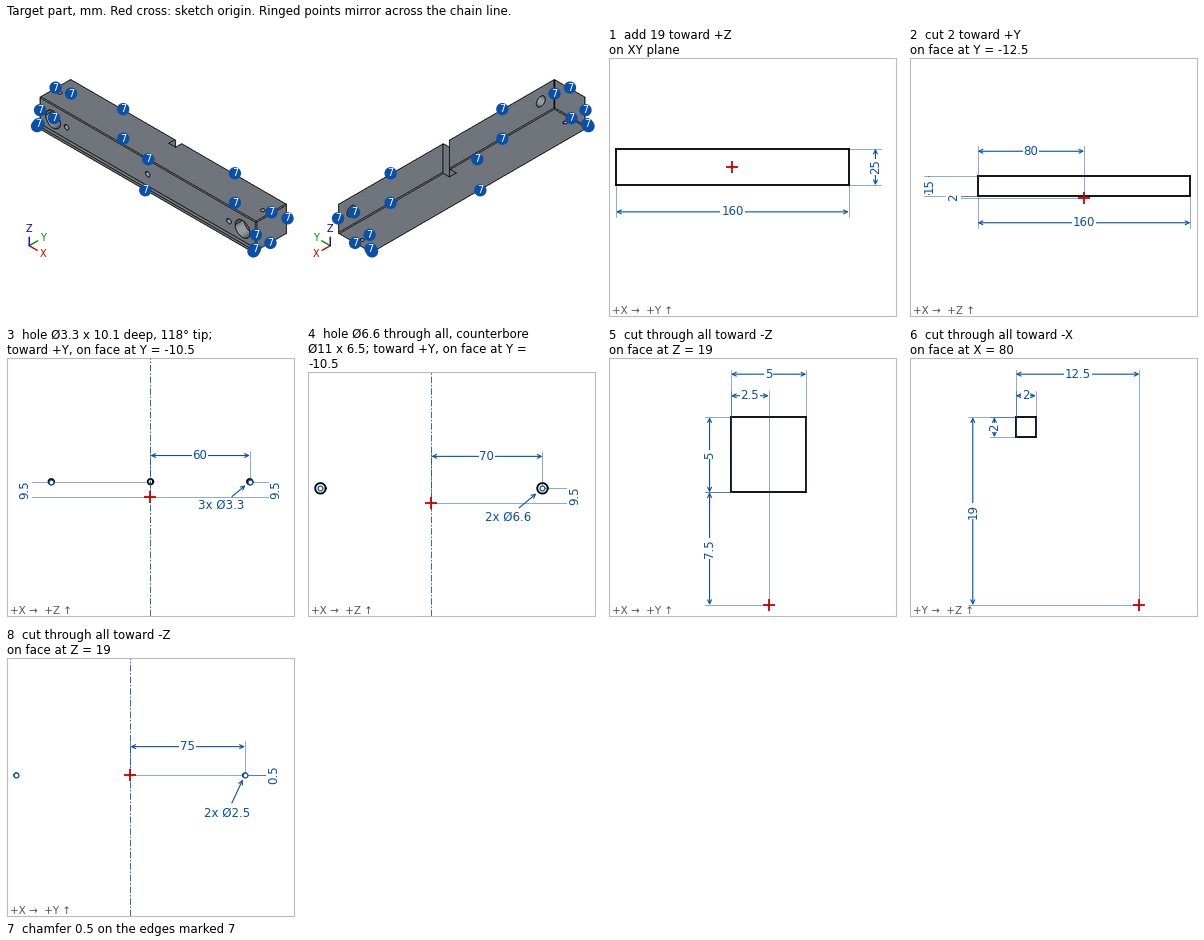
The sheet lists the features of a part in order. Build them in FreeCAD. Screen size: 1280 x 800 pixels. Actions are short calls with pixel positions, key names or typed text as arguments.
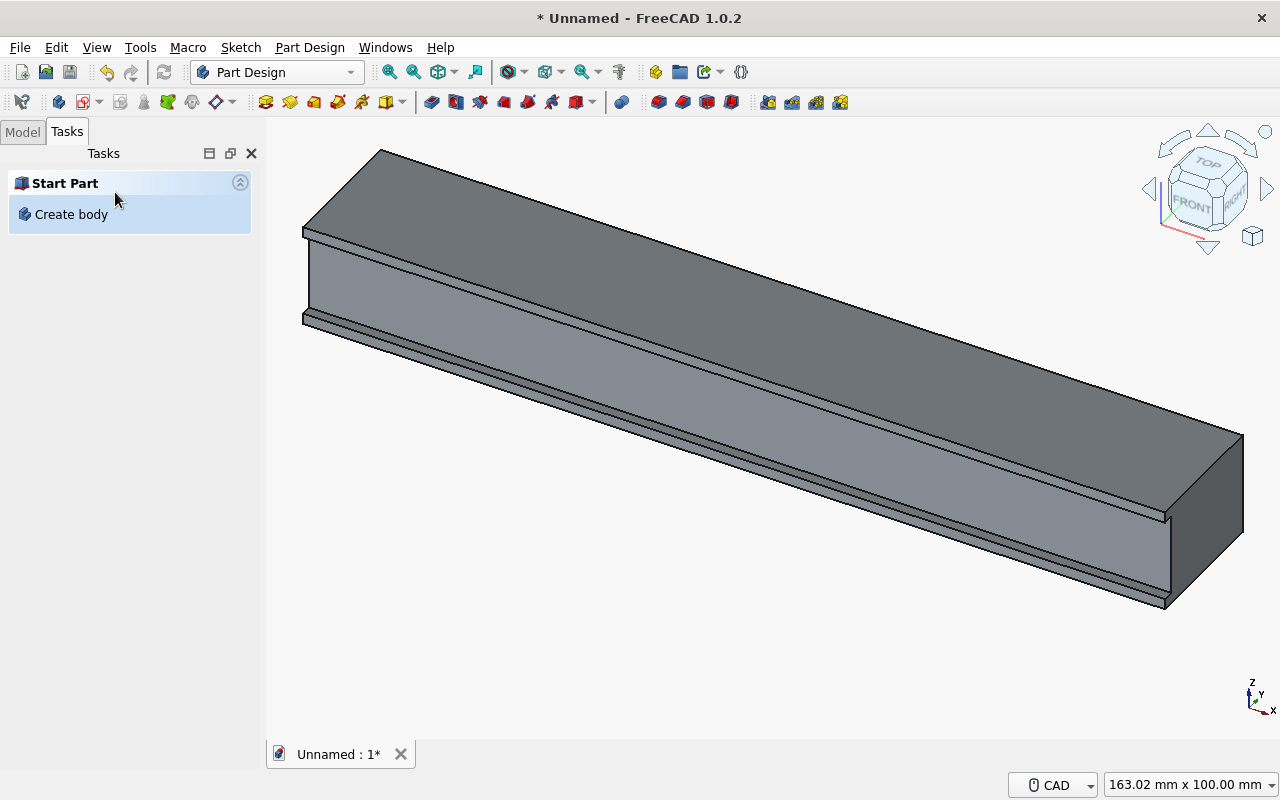
click(1110, 533)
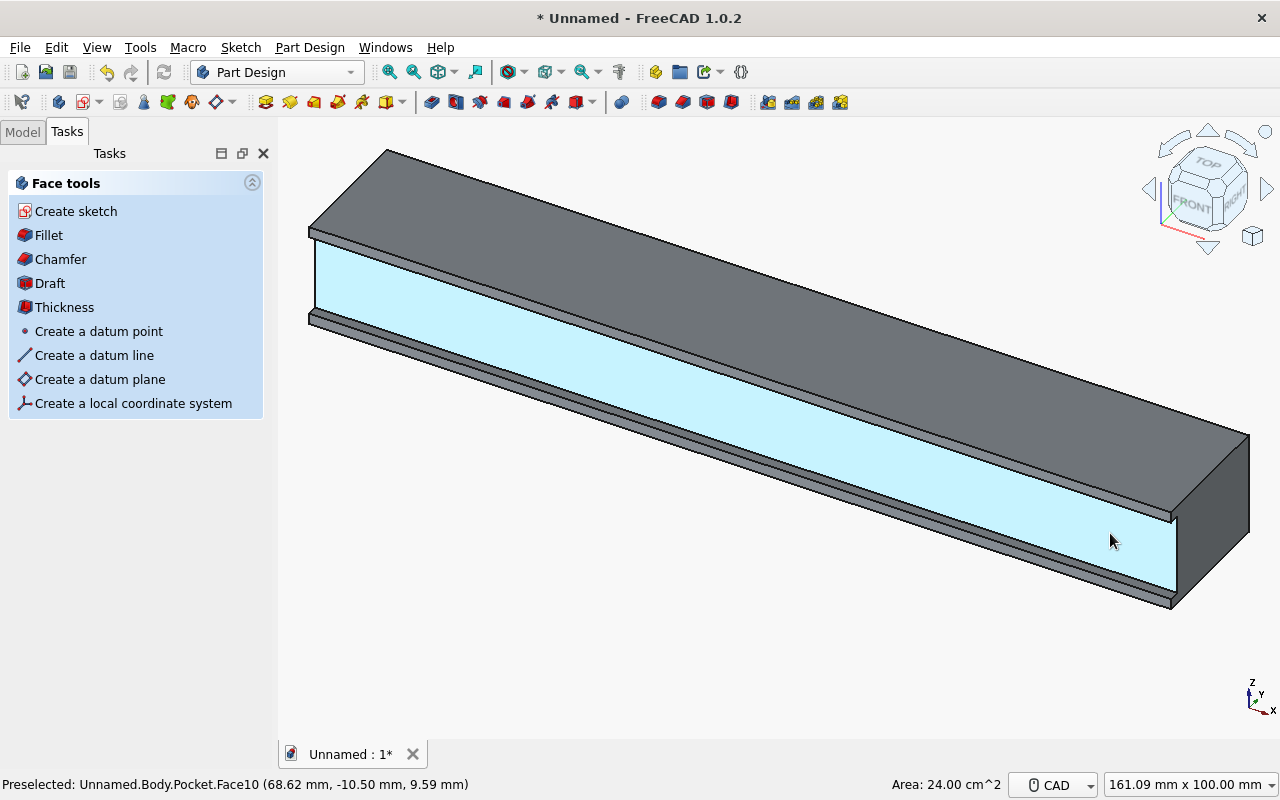
click(84, 102)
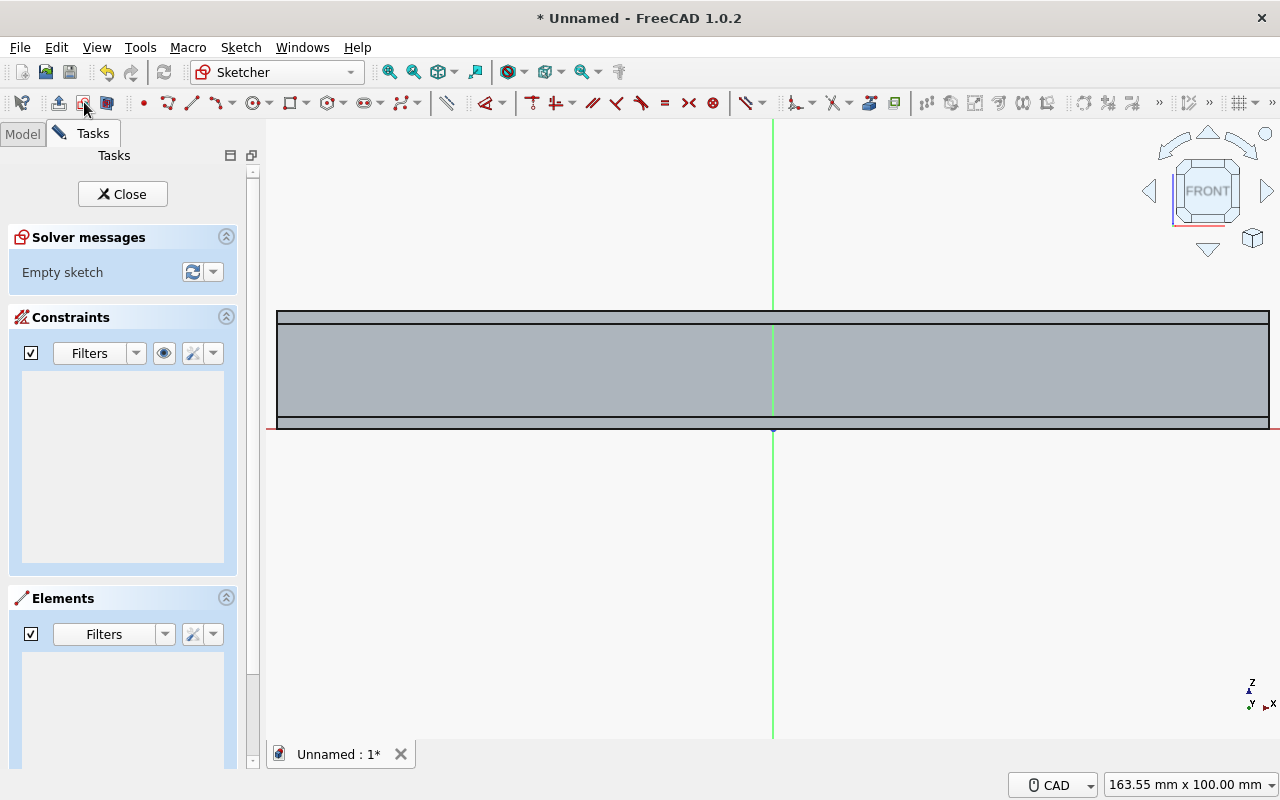
scroll(395, 585, down, 1)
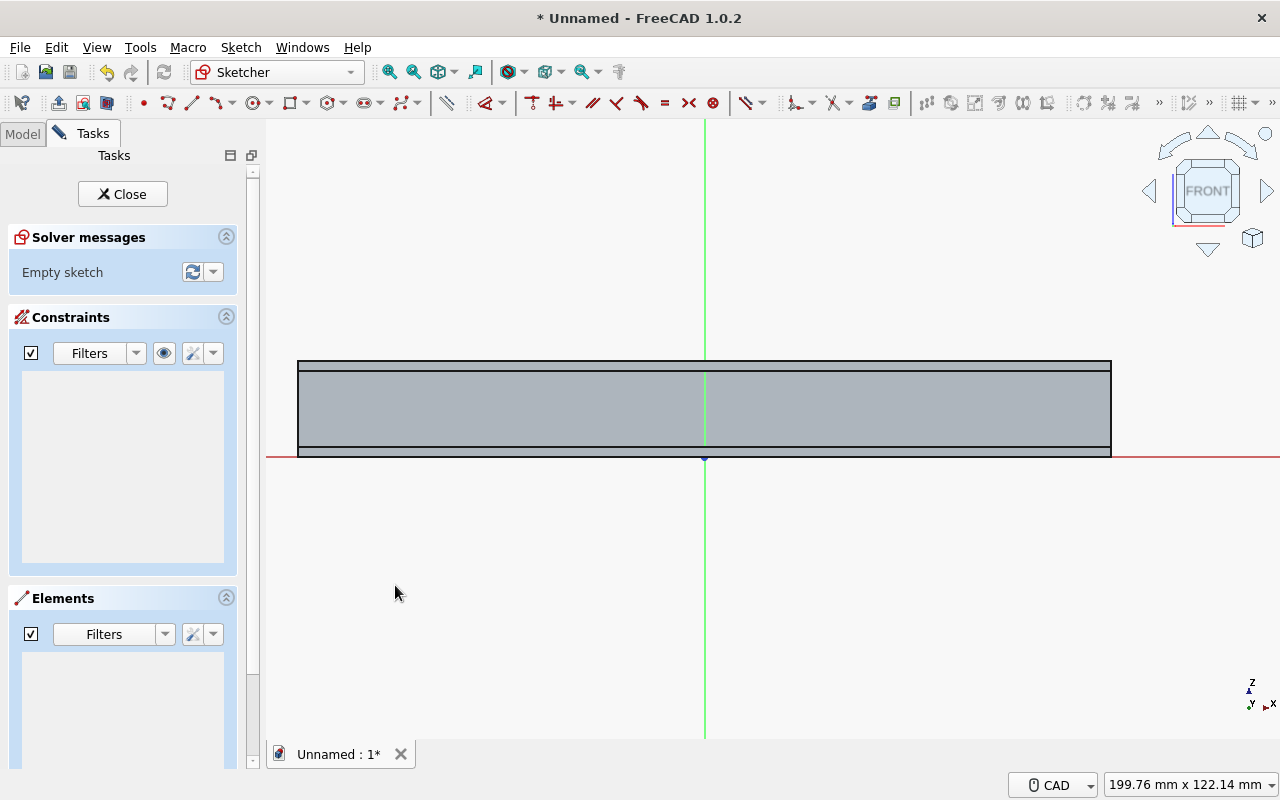
click(254, 104)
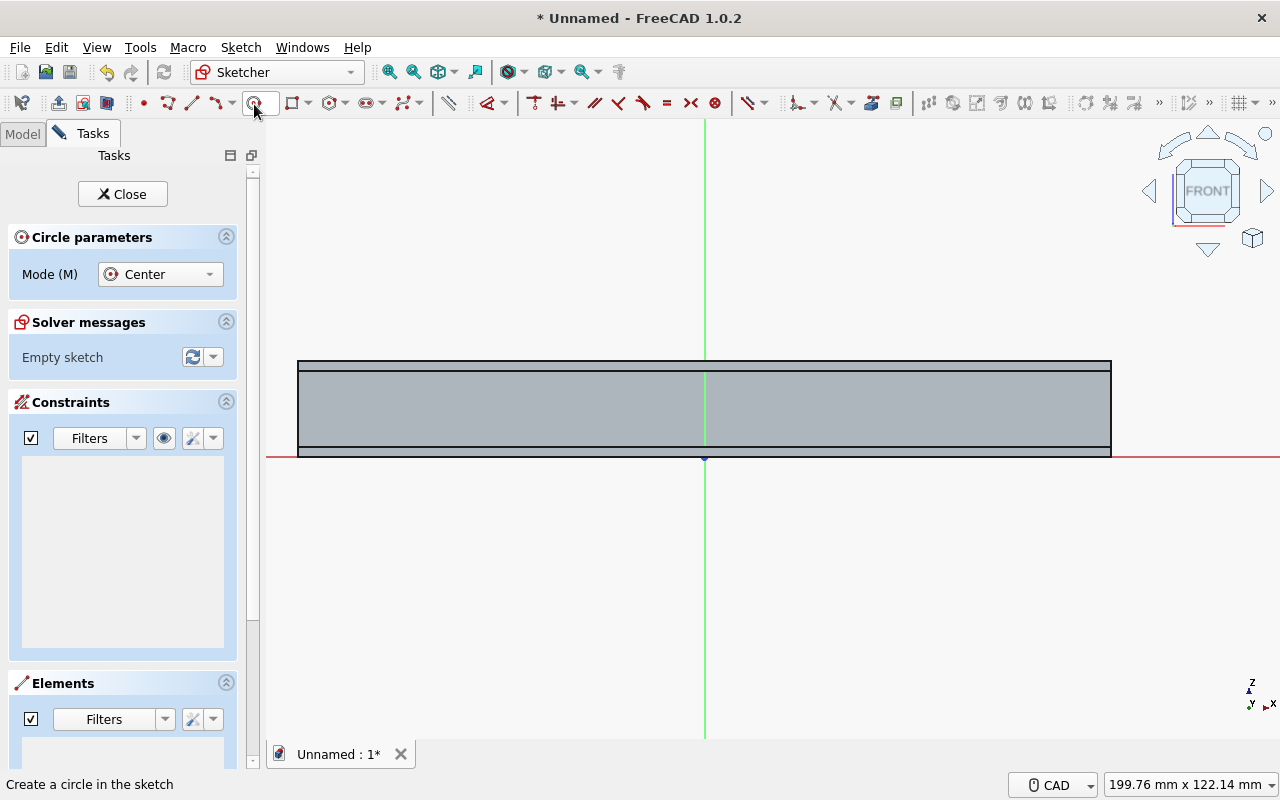
scroll(1009, 409, up, 5)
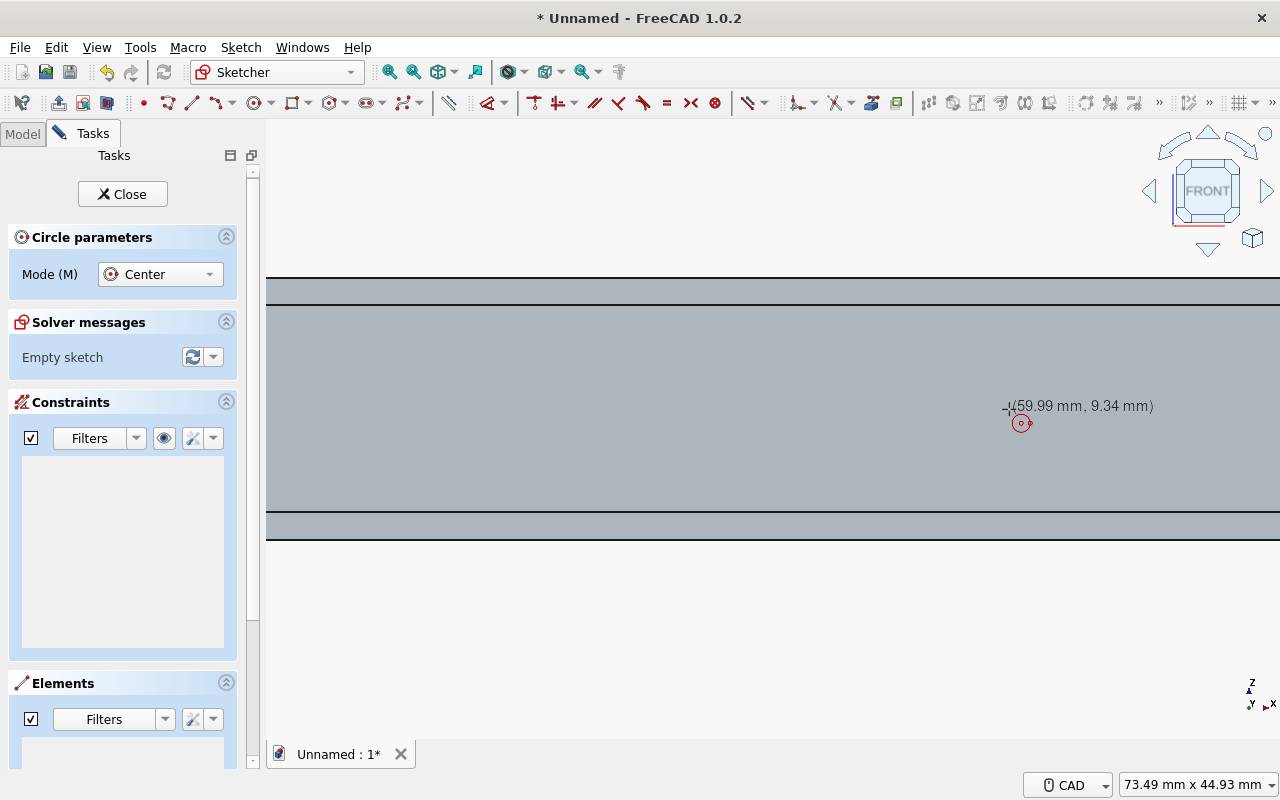
click(1008, 409)
click(1024, 393)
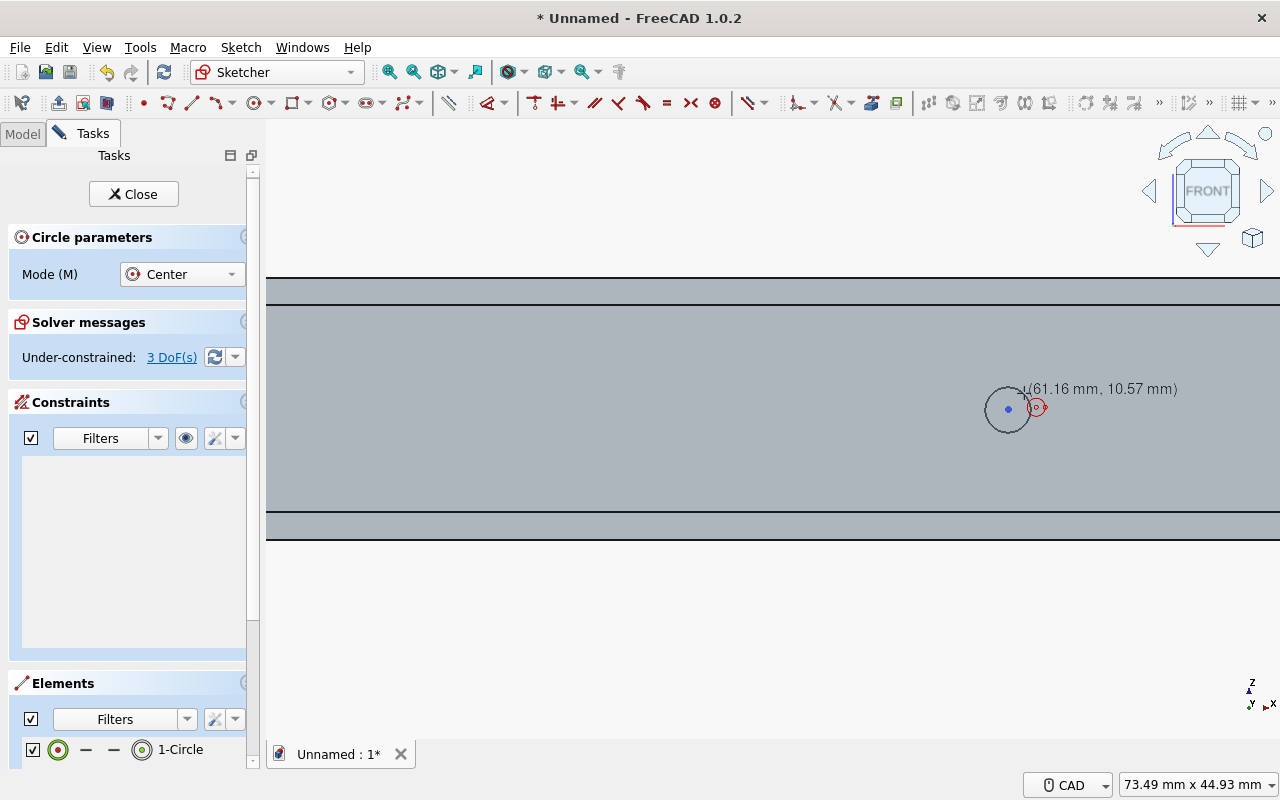
scroll(1010, 409, down, 5)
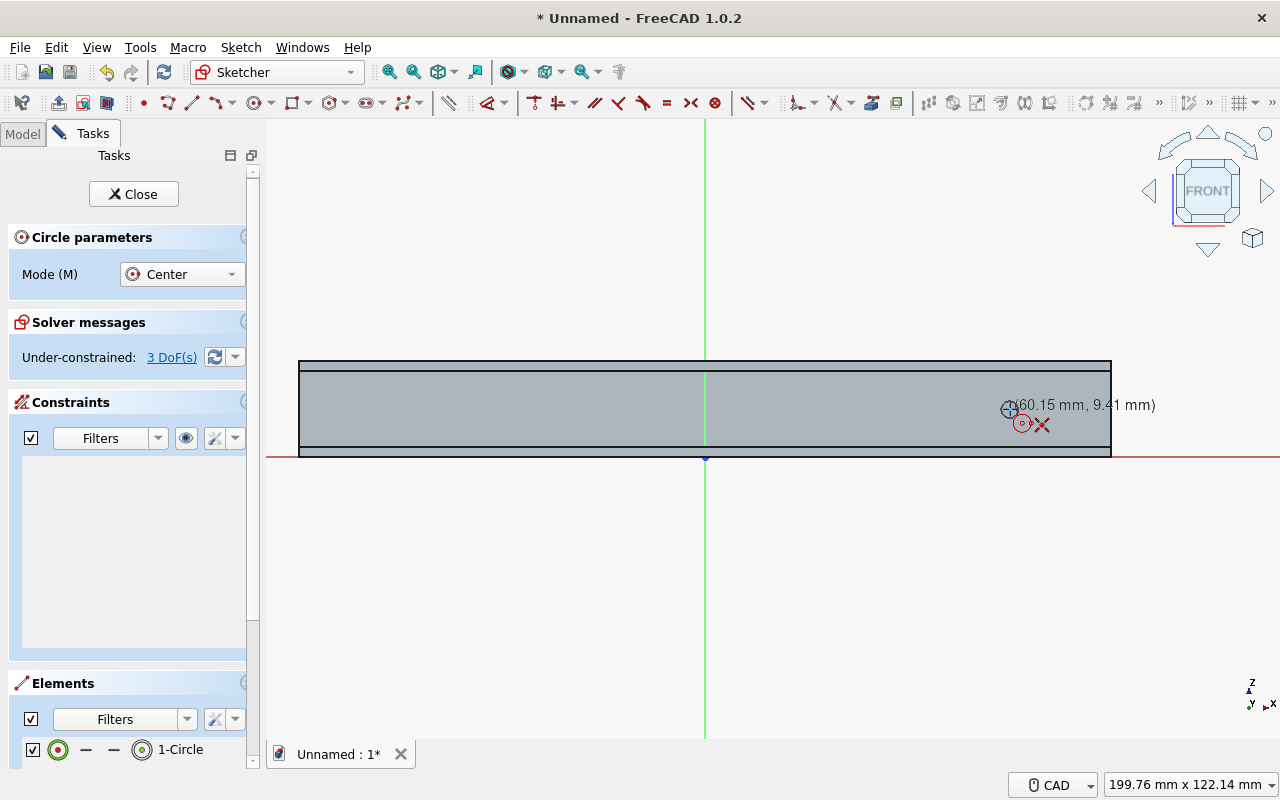
scroll(705, 409, up, 5)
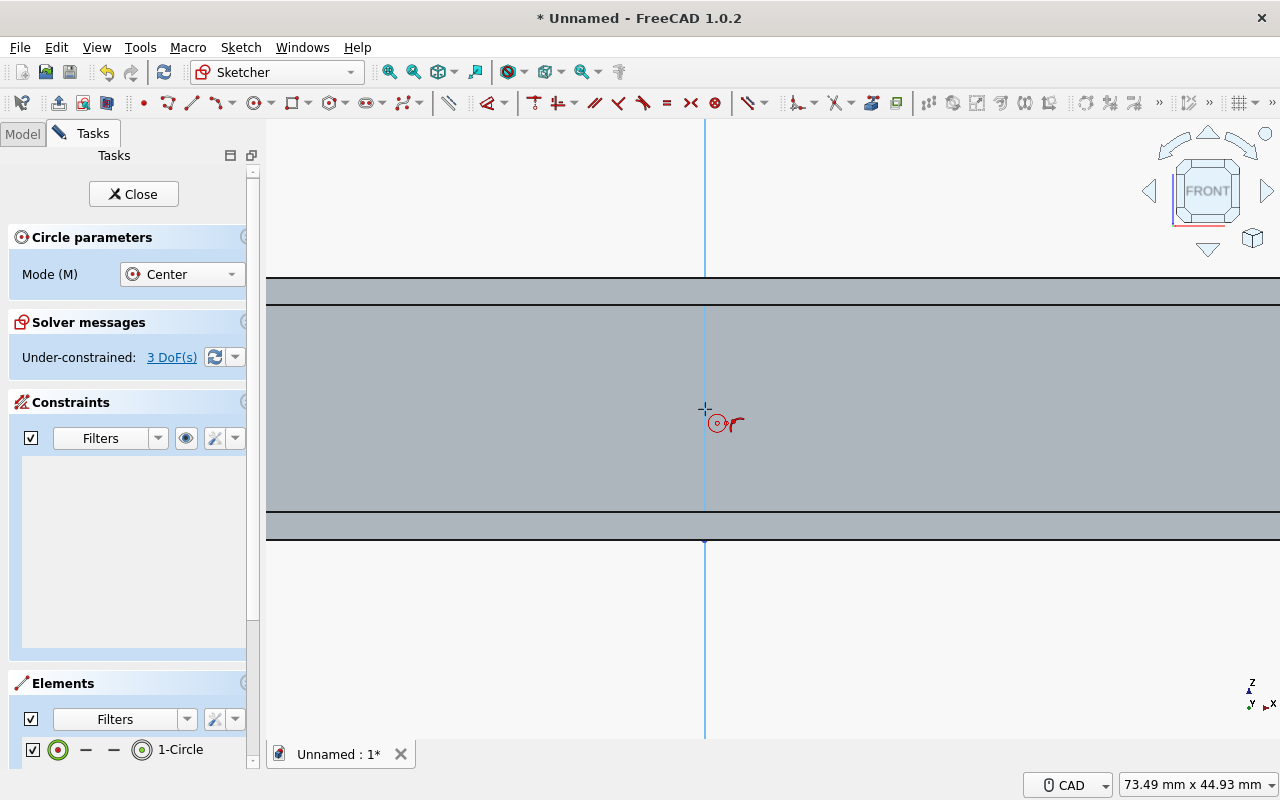
click(705, 409)
click(721, 393)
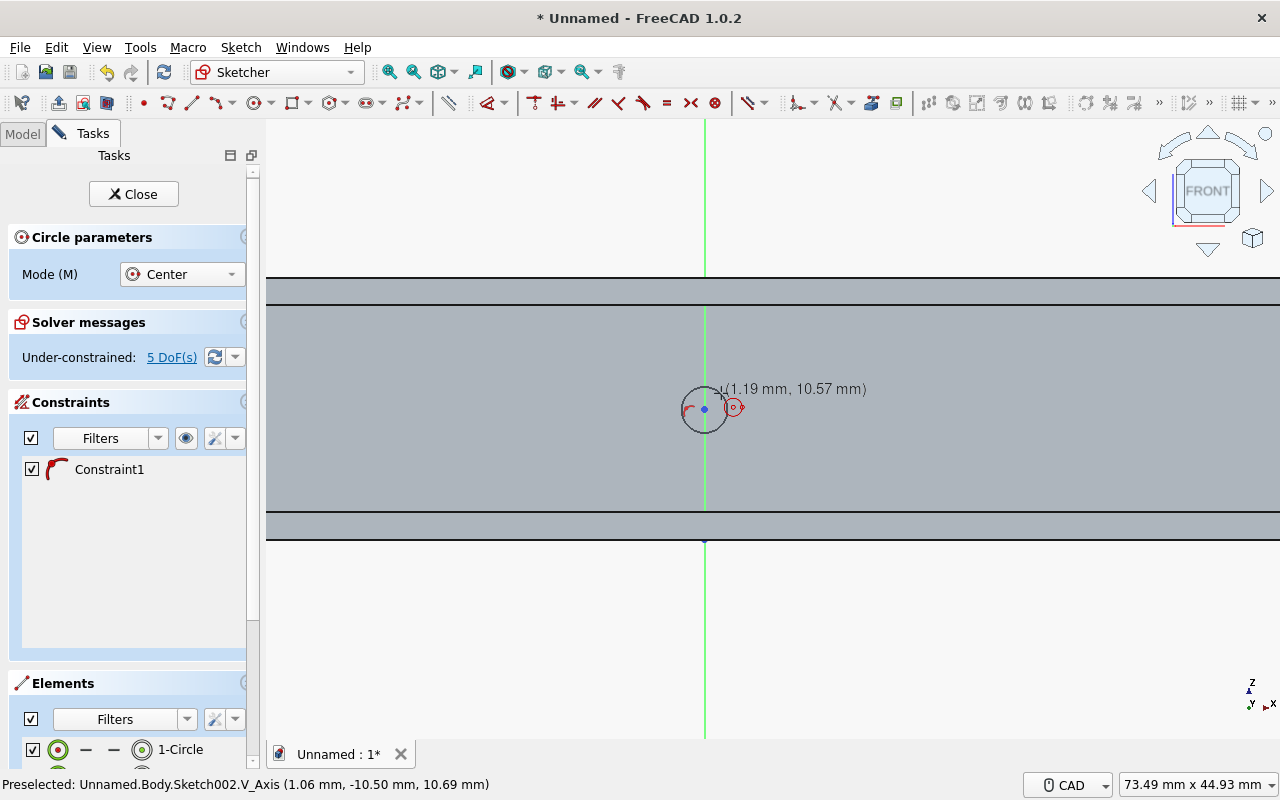
scroll(704, 409, down, 5)